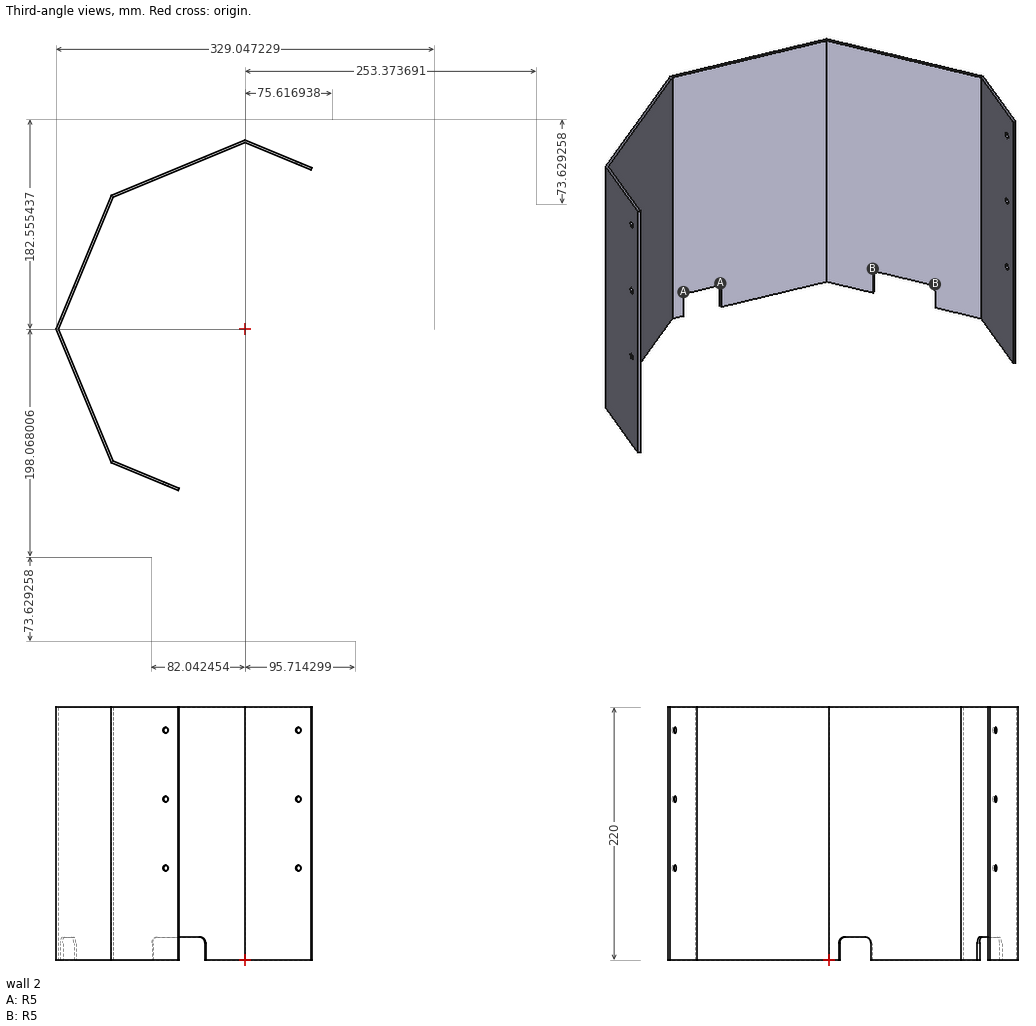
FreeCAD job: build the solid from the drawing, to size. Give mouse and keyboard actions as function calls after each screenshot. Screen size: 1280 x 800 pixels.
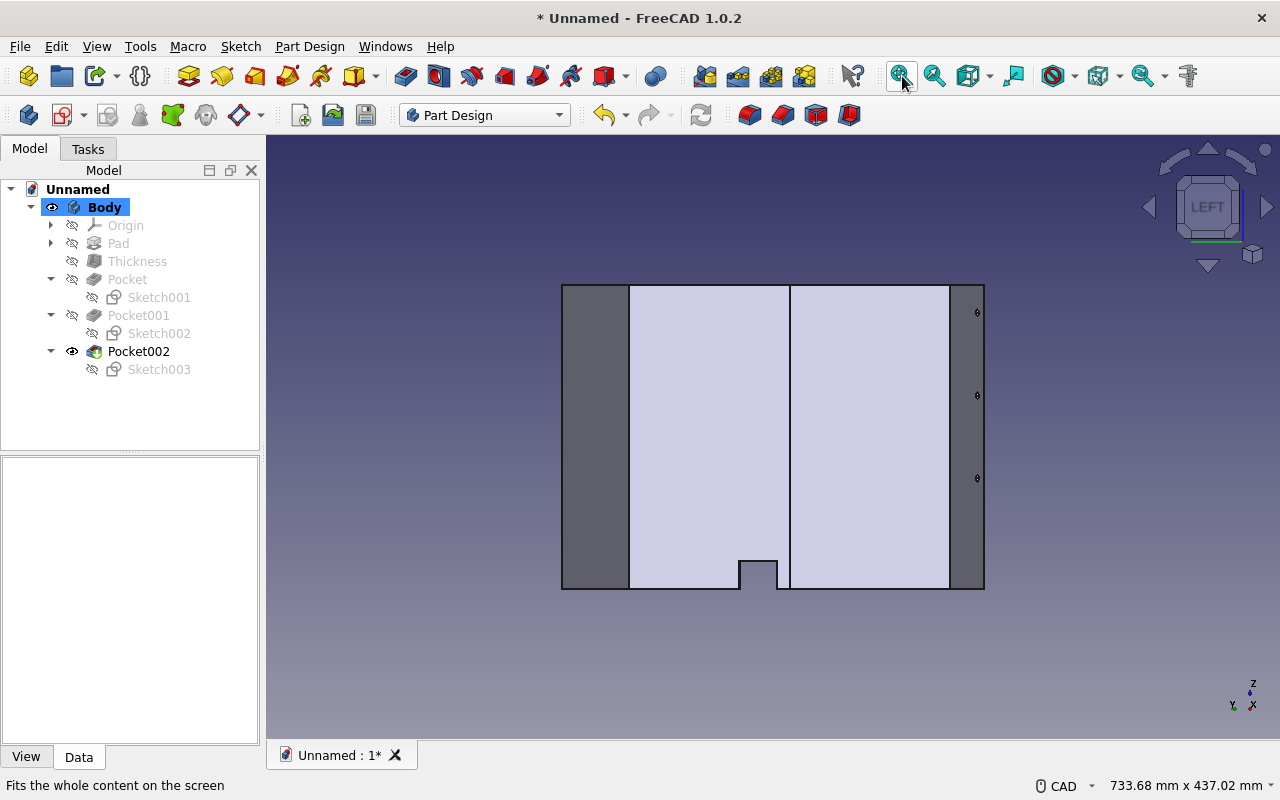
key(v)
key(3)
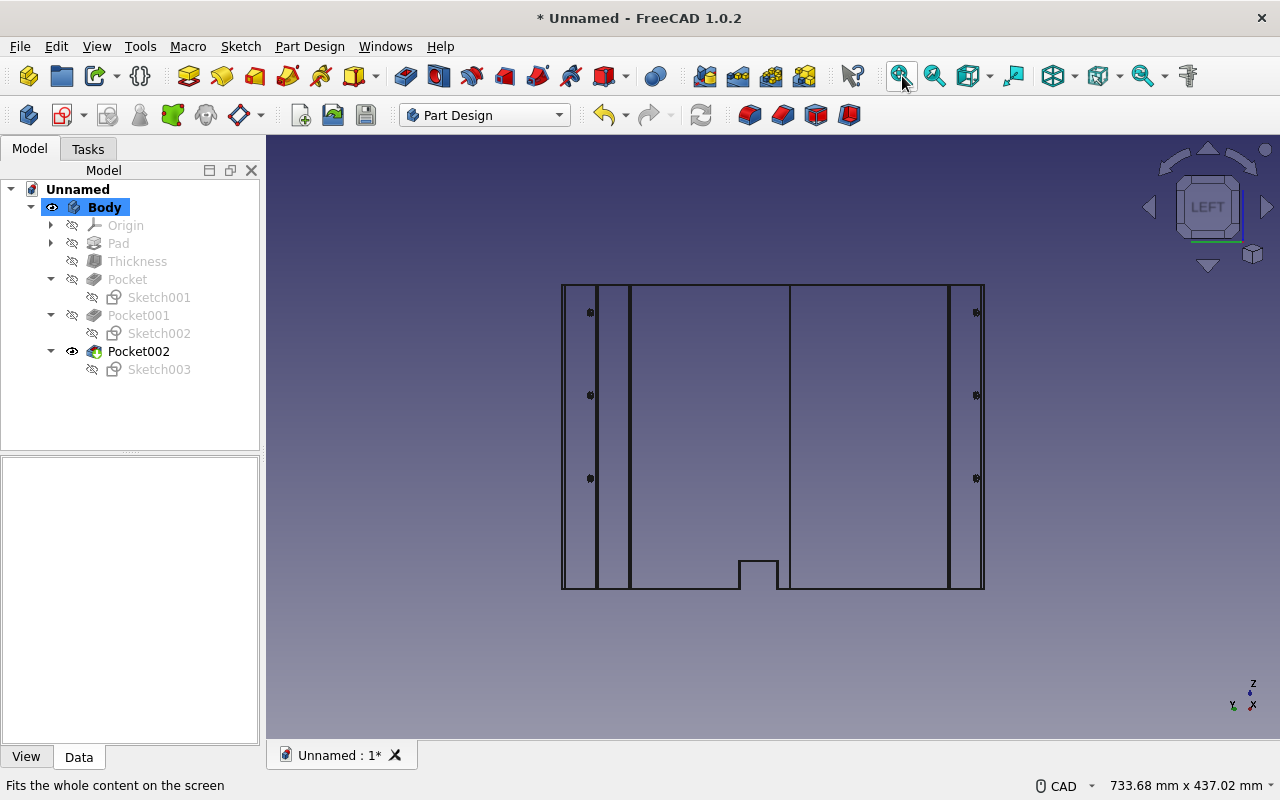
key(0)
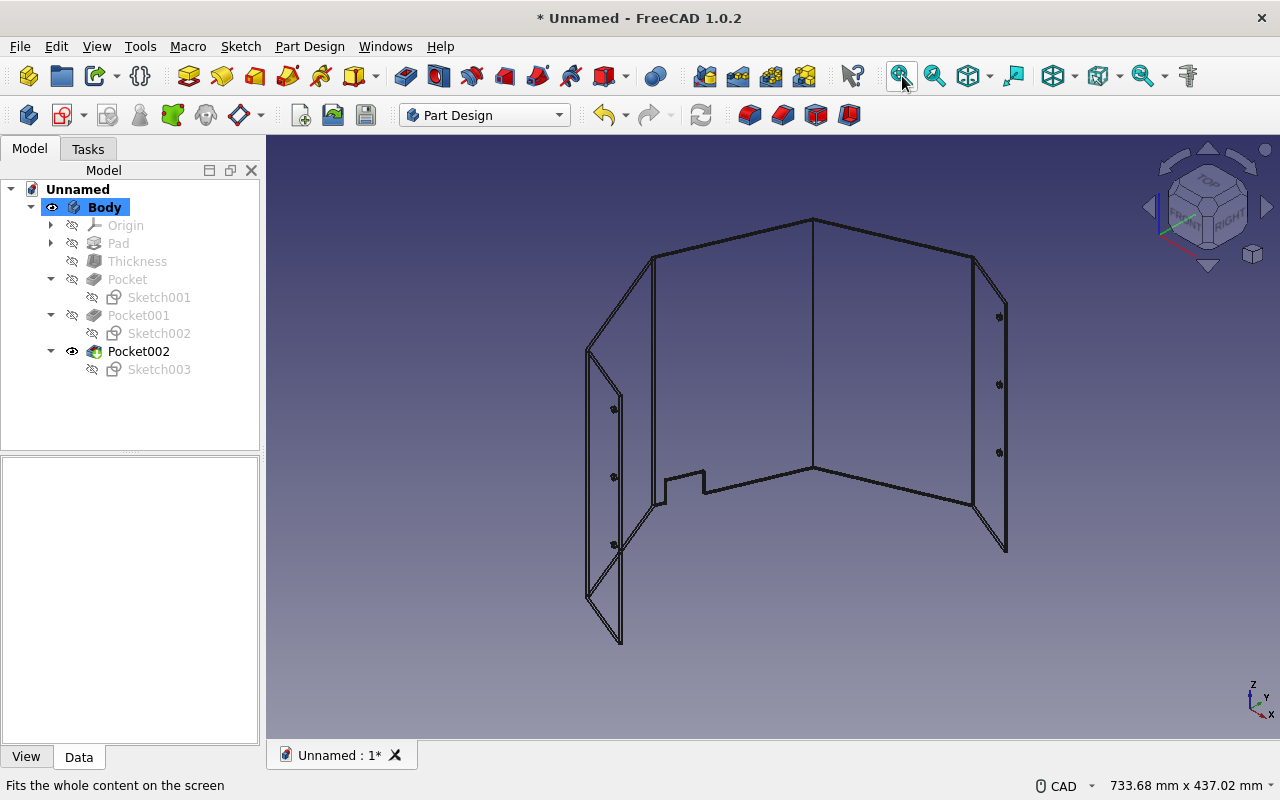
scroll(704, 470, up, 14)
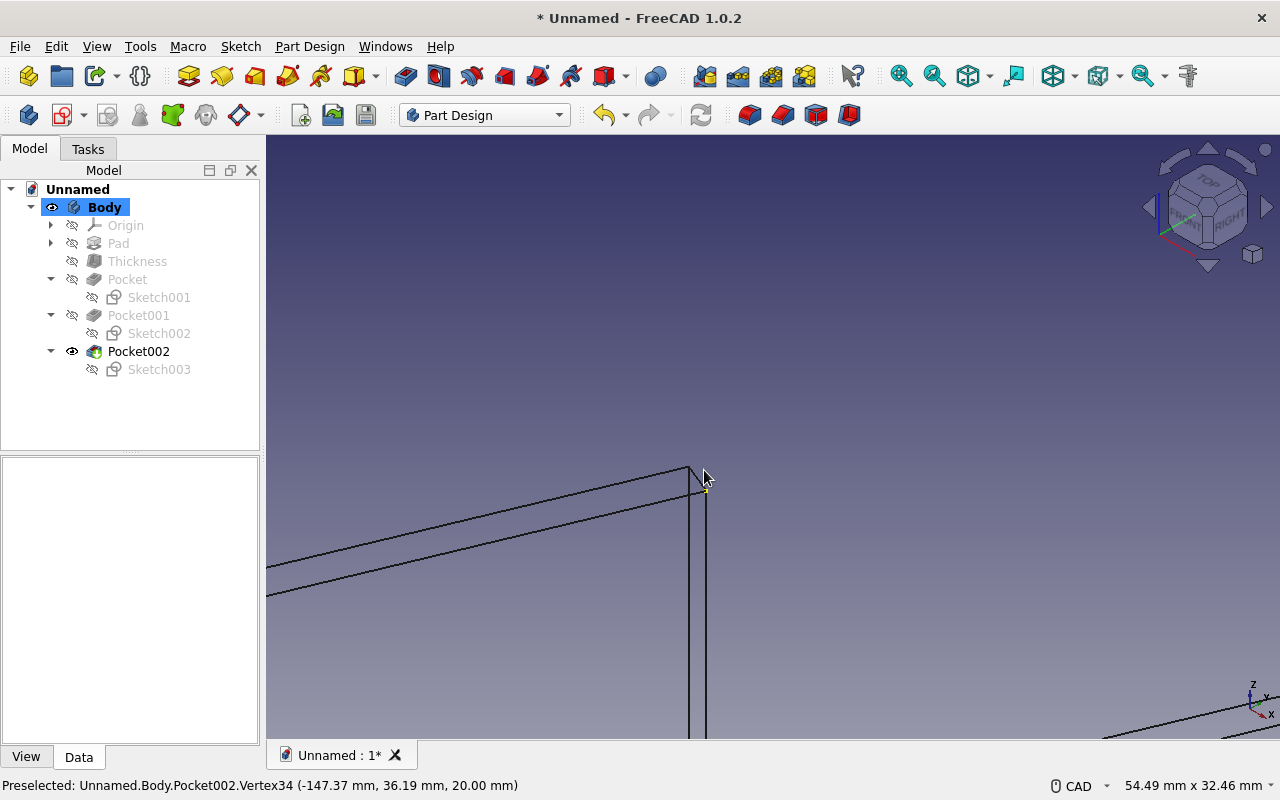
click(698, 478)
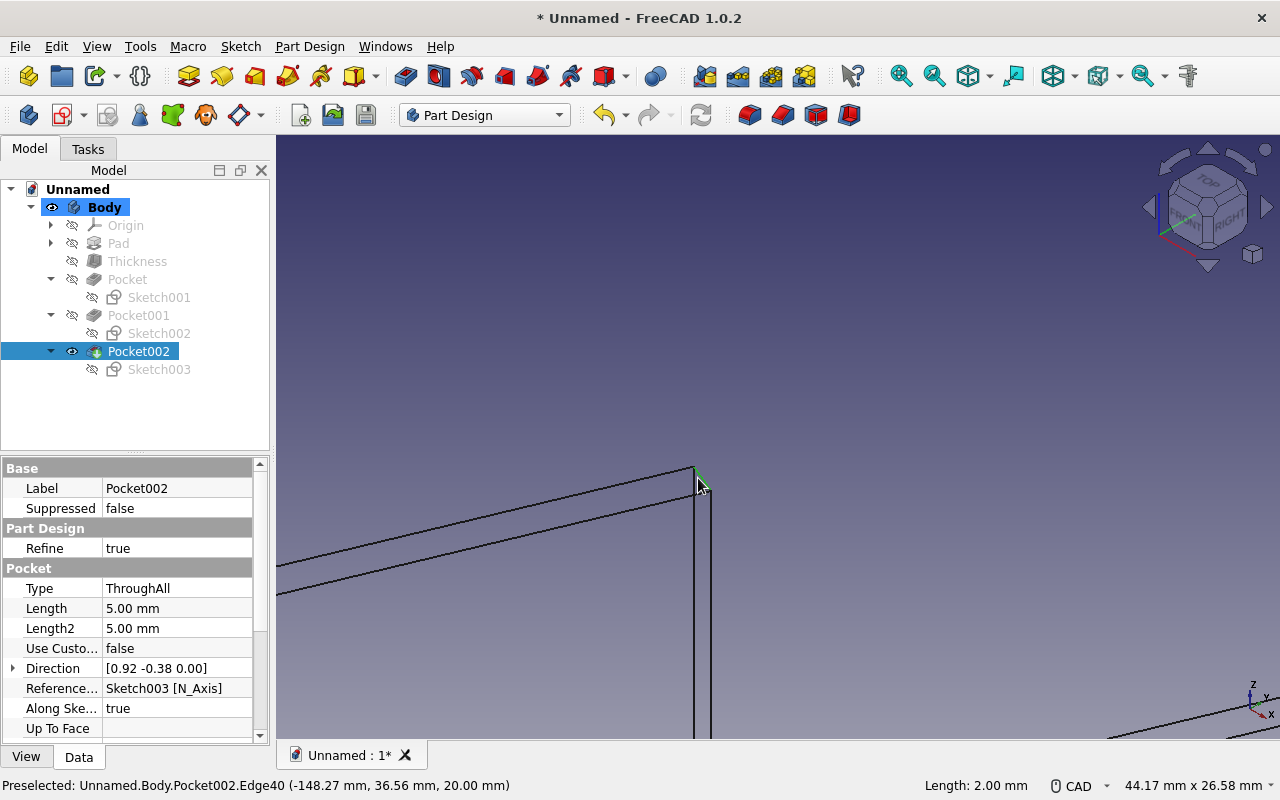
click(902, 76)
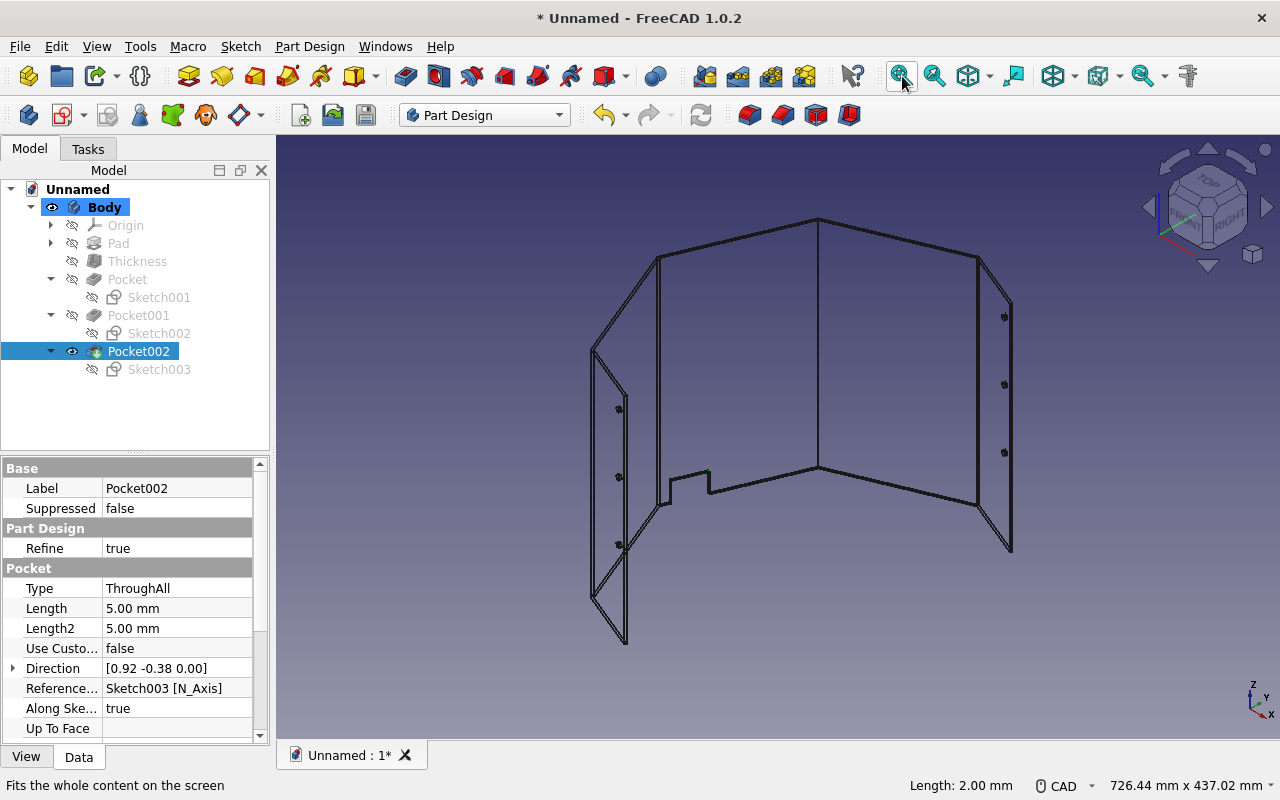
key(2)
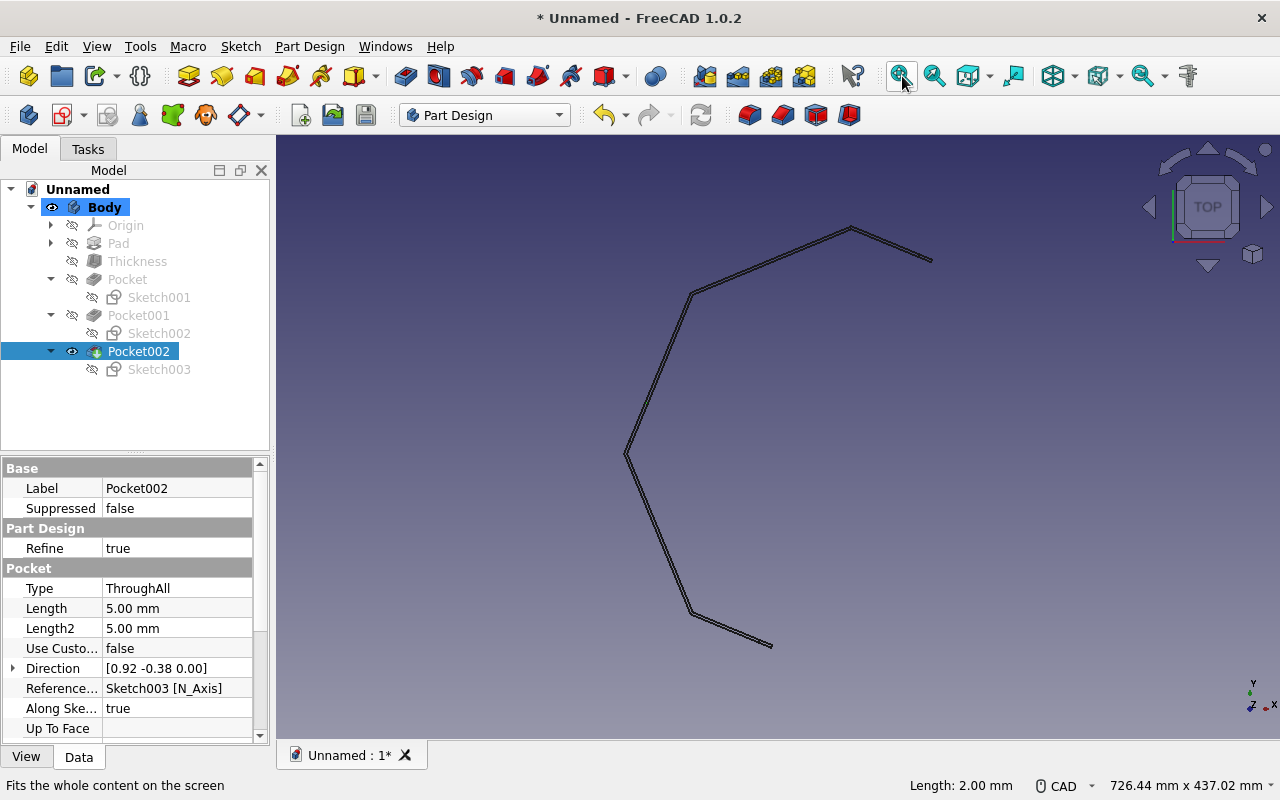
scroll(631, 440, up, 14)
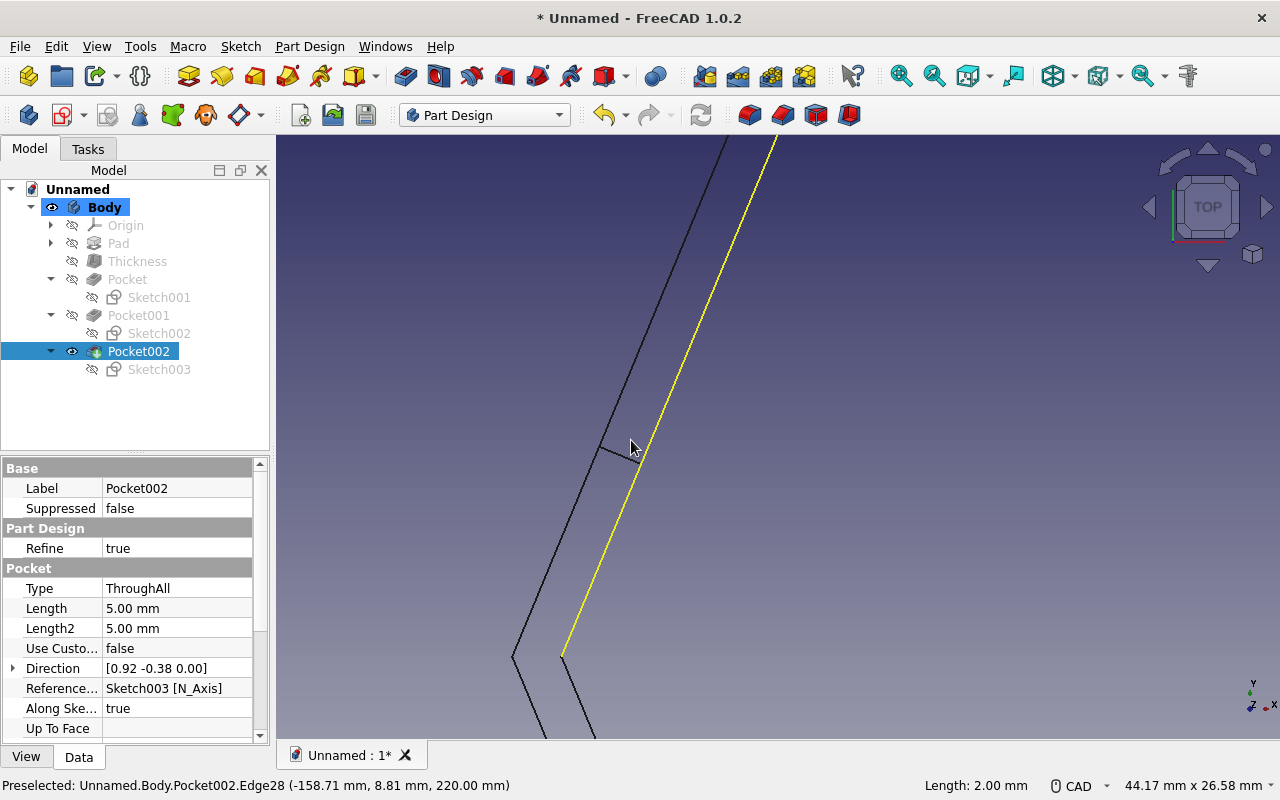
click(620, 454, ctrl)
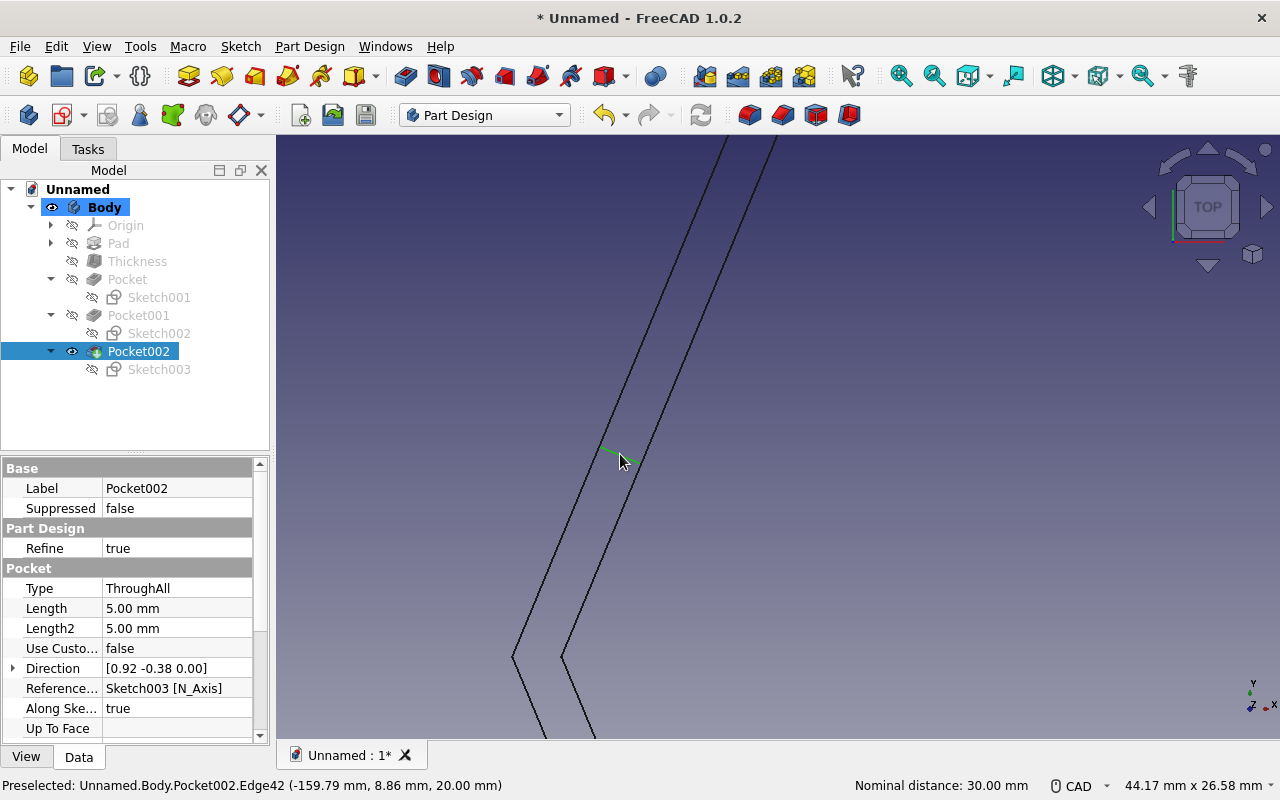
key(v)
key(1)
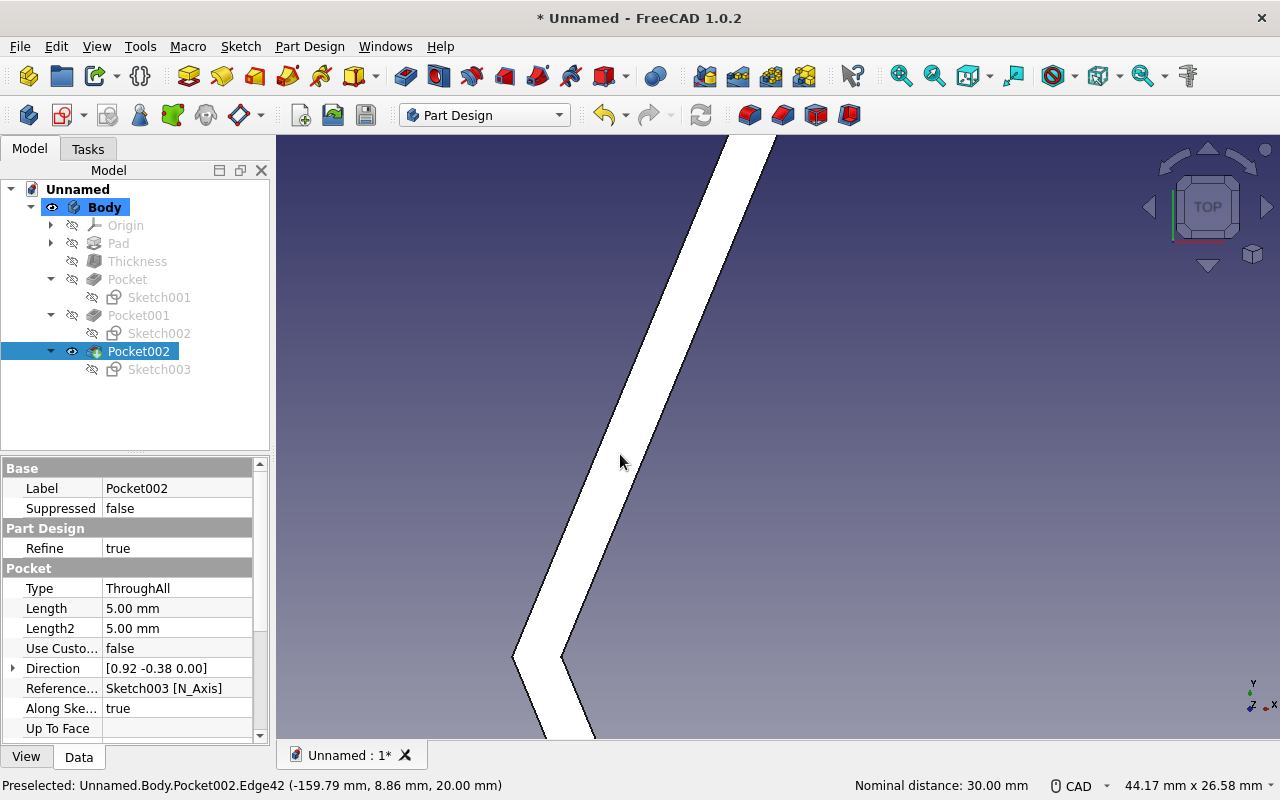
click(750, 116)